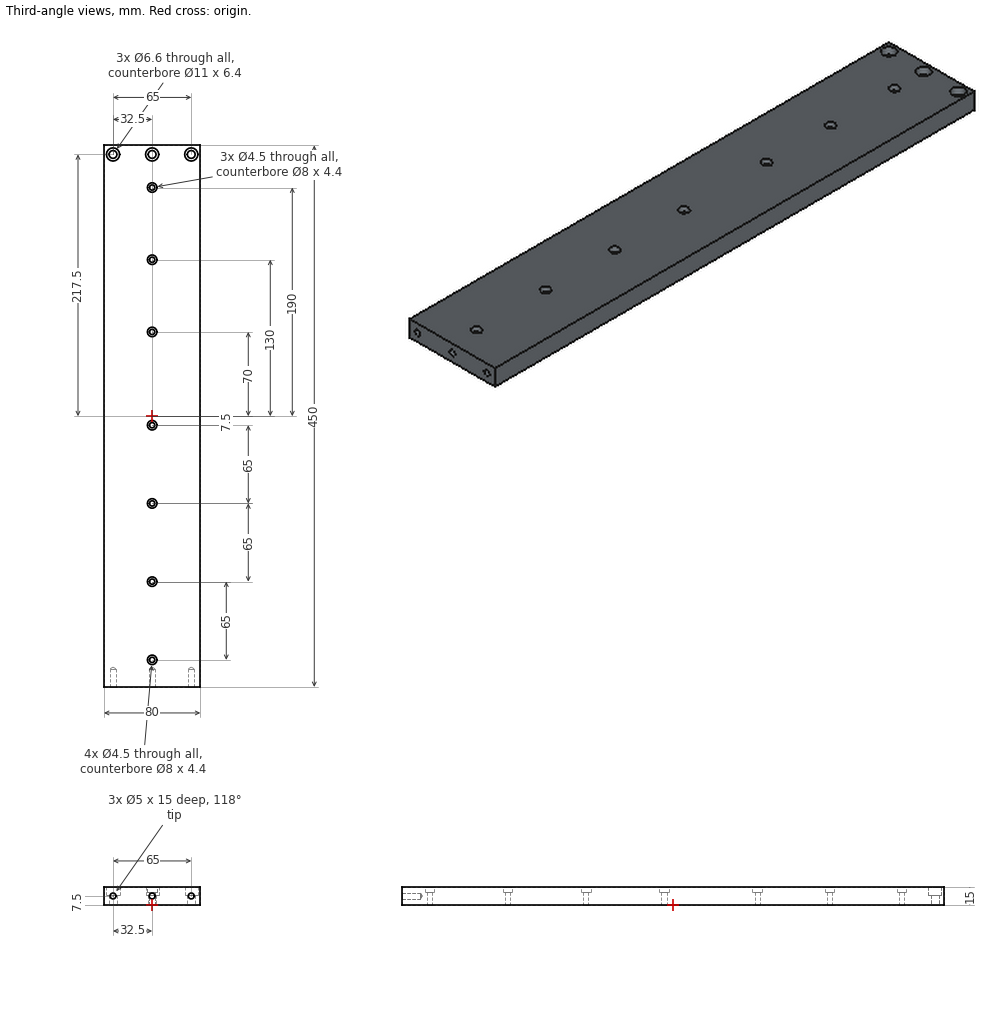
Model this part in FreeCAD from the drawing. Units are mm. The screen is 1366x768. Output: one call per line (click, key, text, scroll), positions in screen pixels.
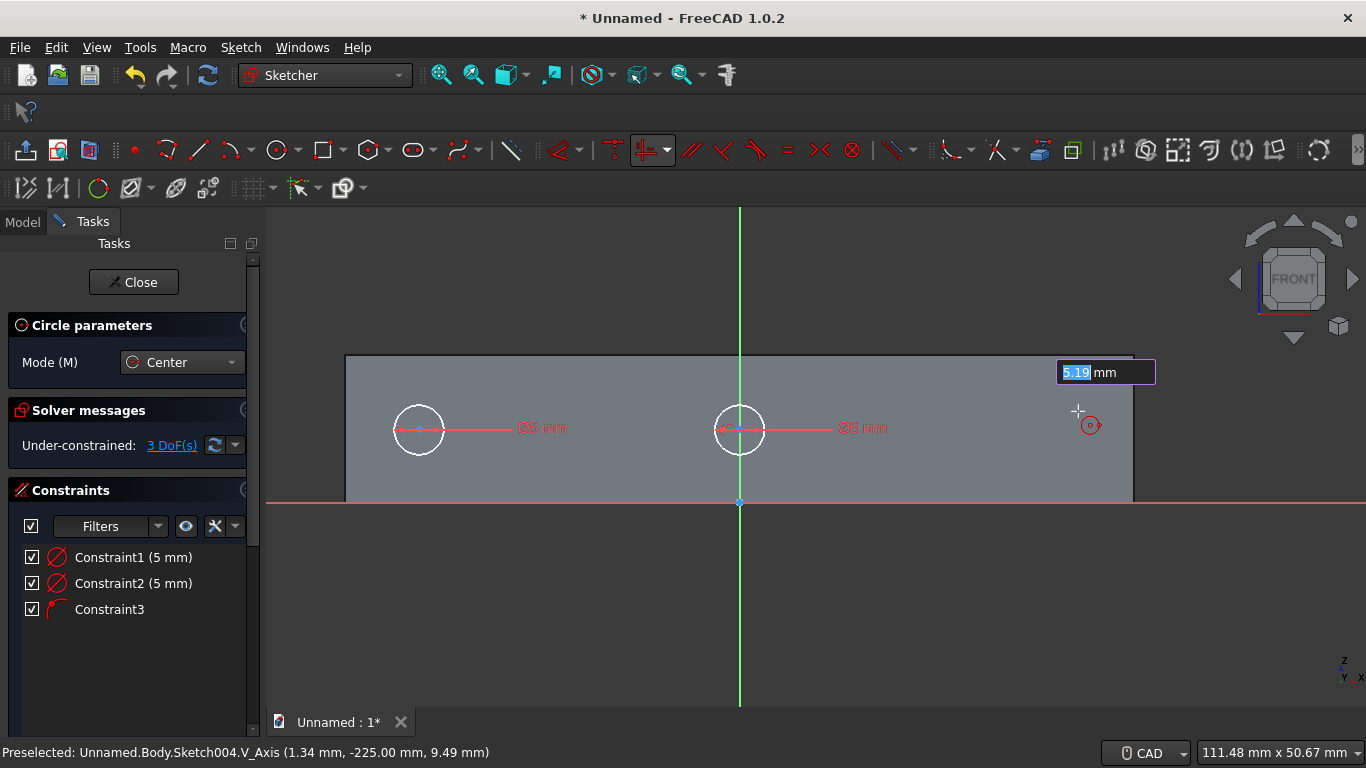
text(5)
key(Return)
key(Escape)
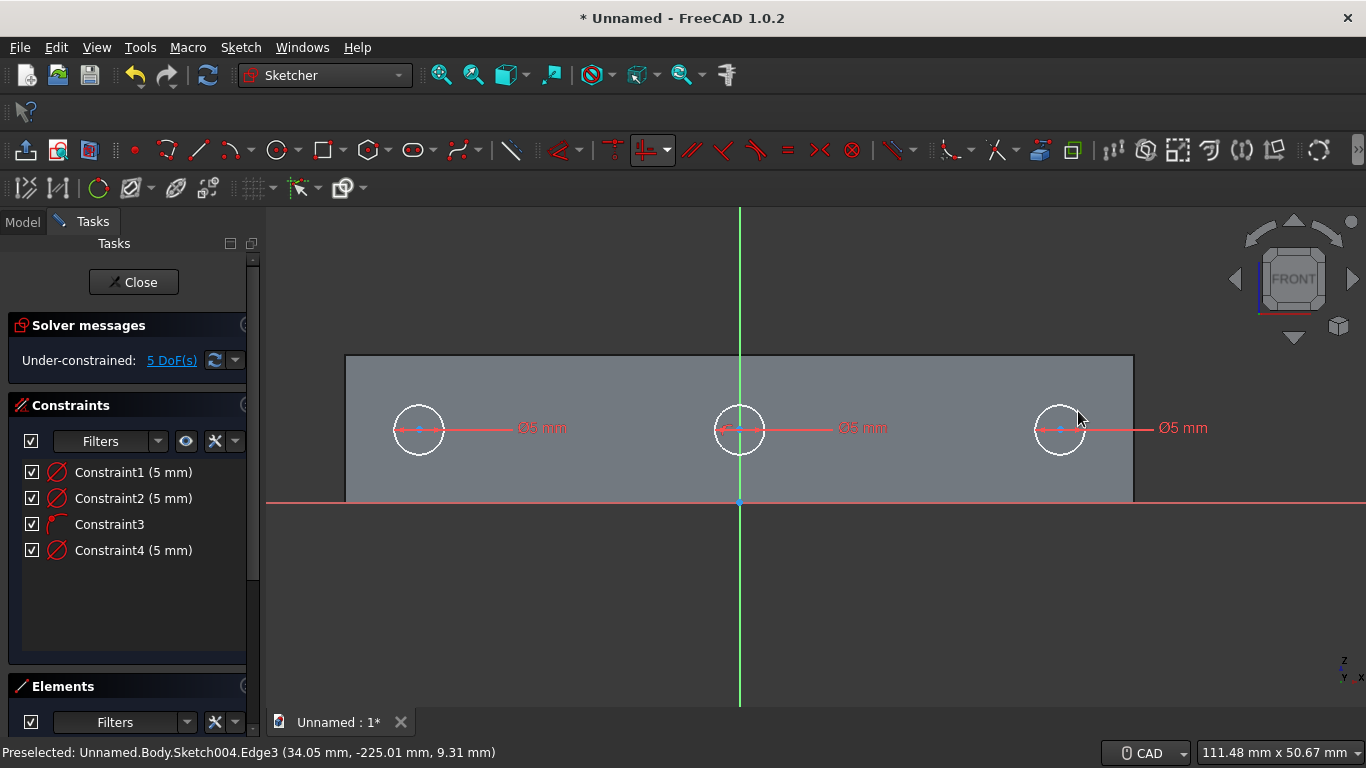
click(419, 430)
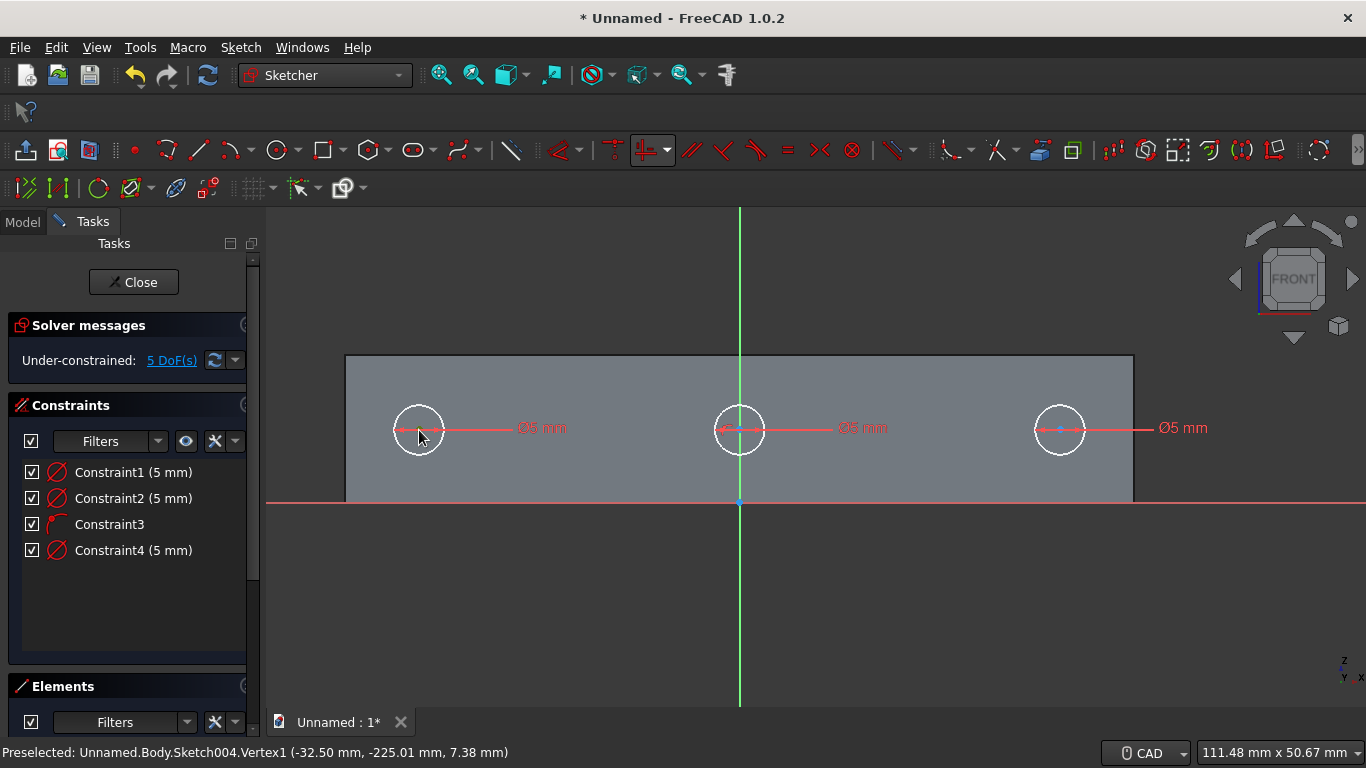
click(740, 430)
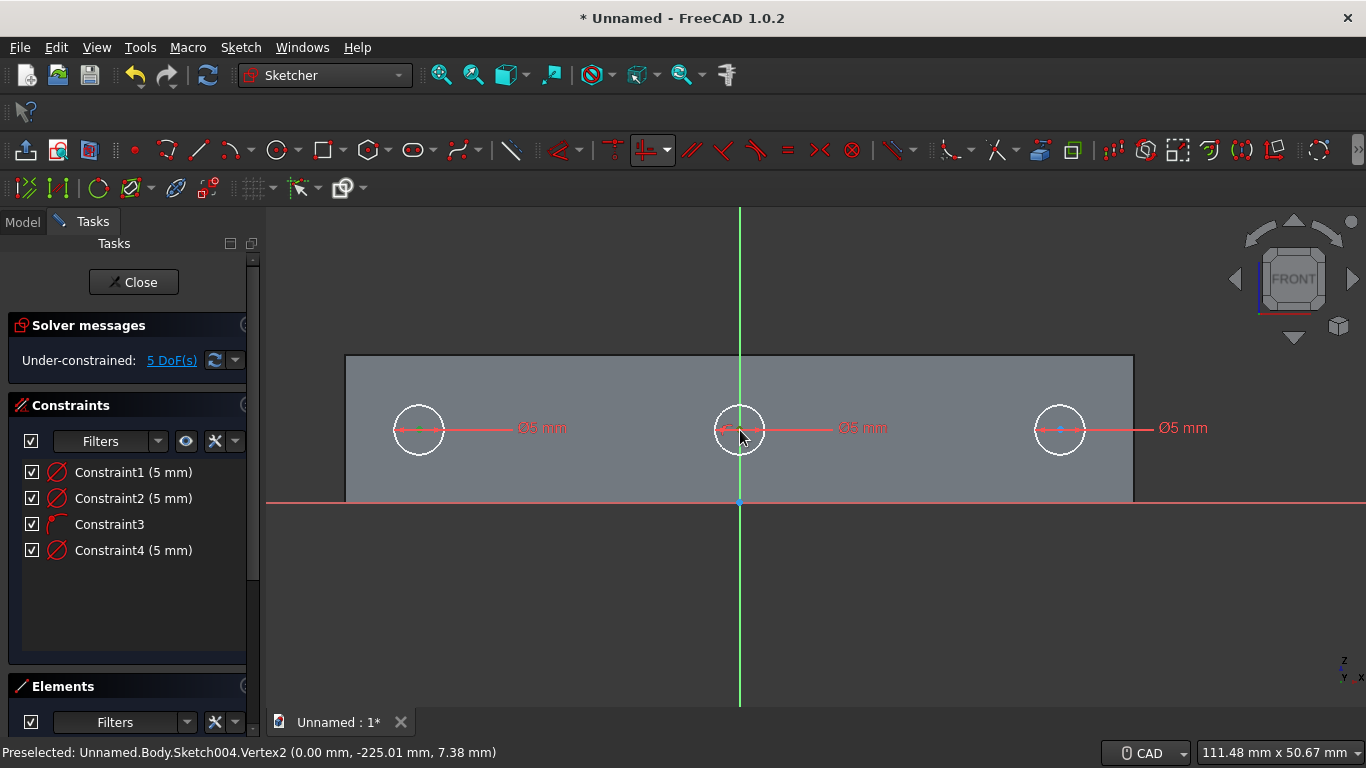
key(h)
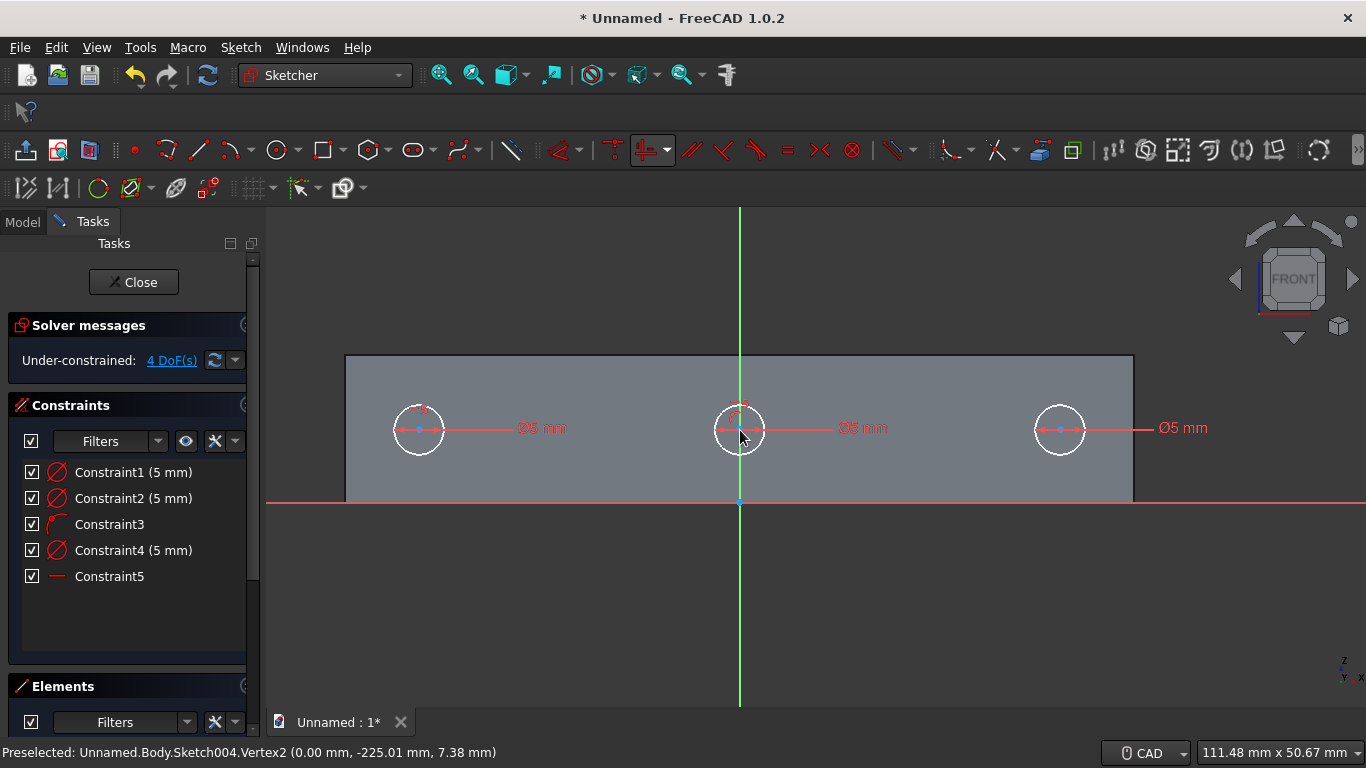
click(740, 430)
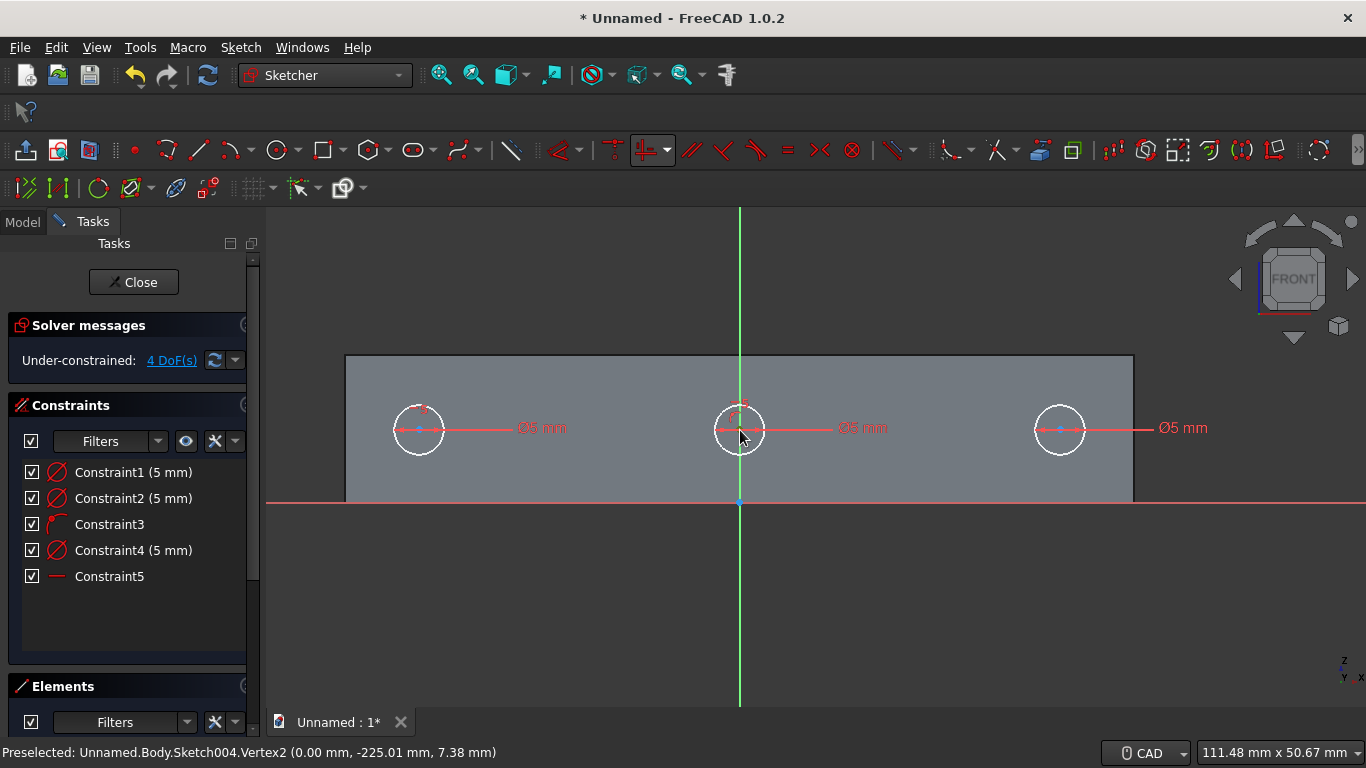
click(1060, 430)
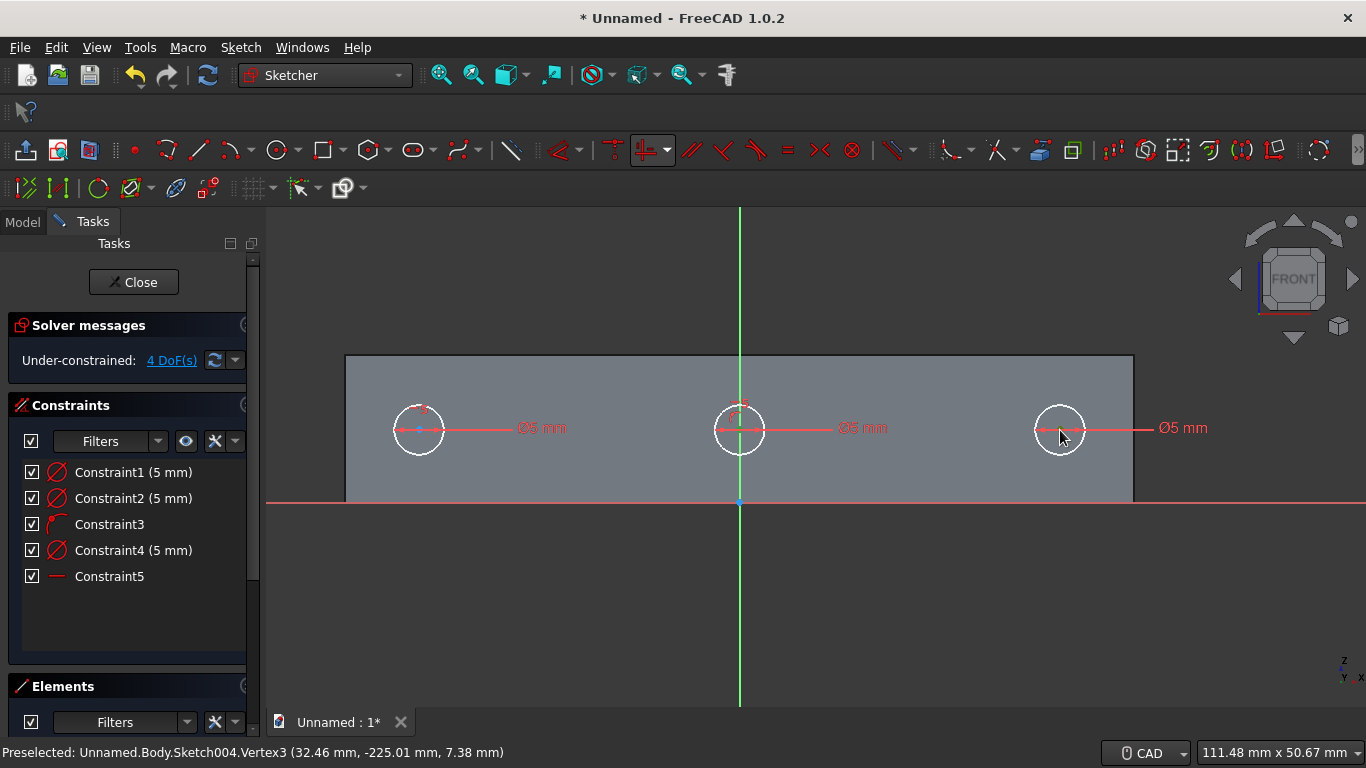
click(670, 150)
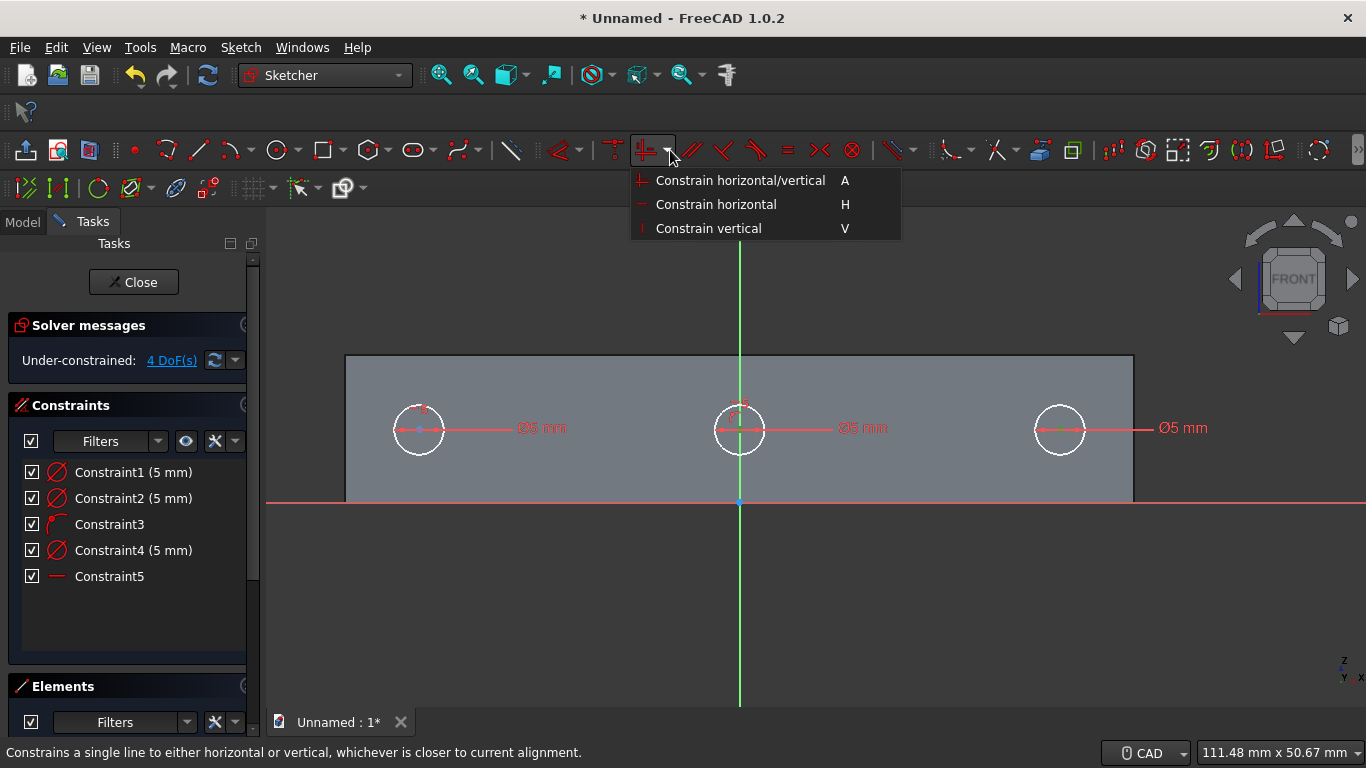
click(766, 204)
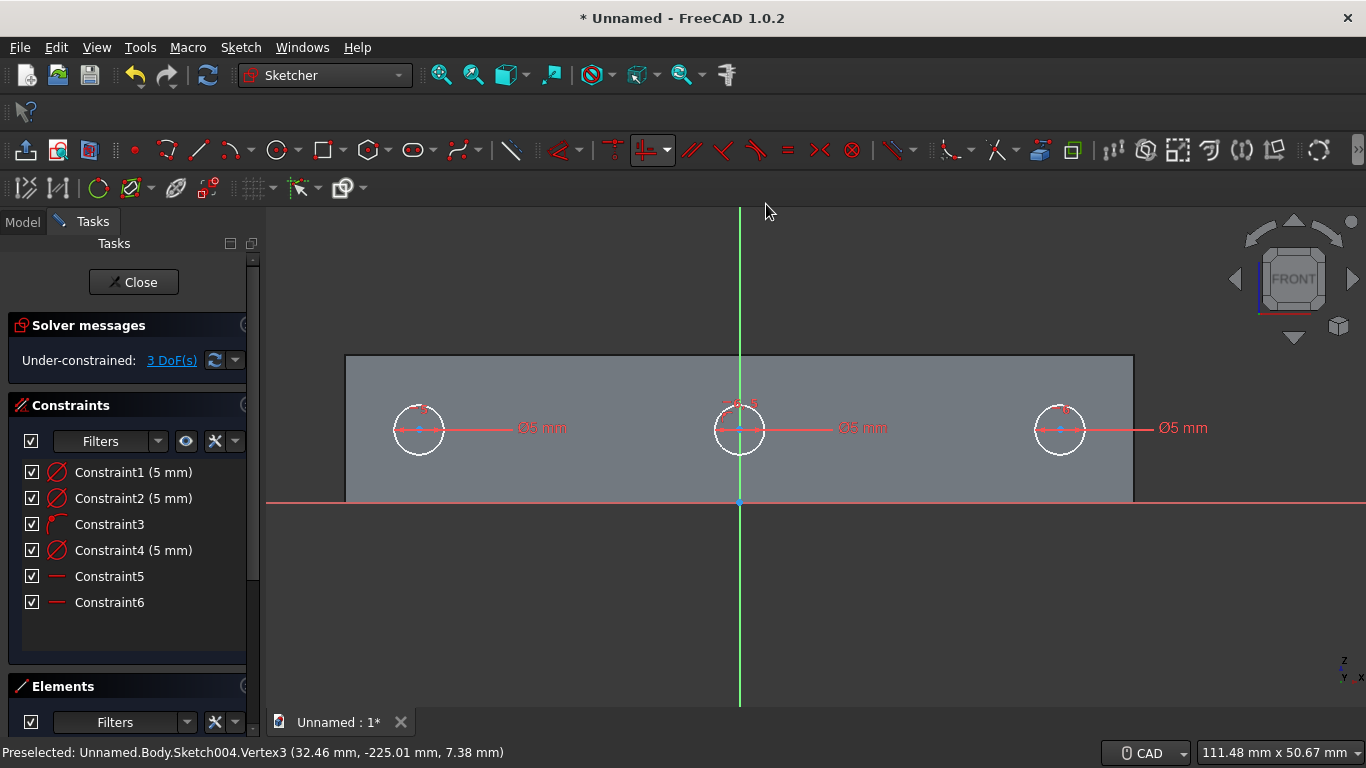
click(558, 150)